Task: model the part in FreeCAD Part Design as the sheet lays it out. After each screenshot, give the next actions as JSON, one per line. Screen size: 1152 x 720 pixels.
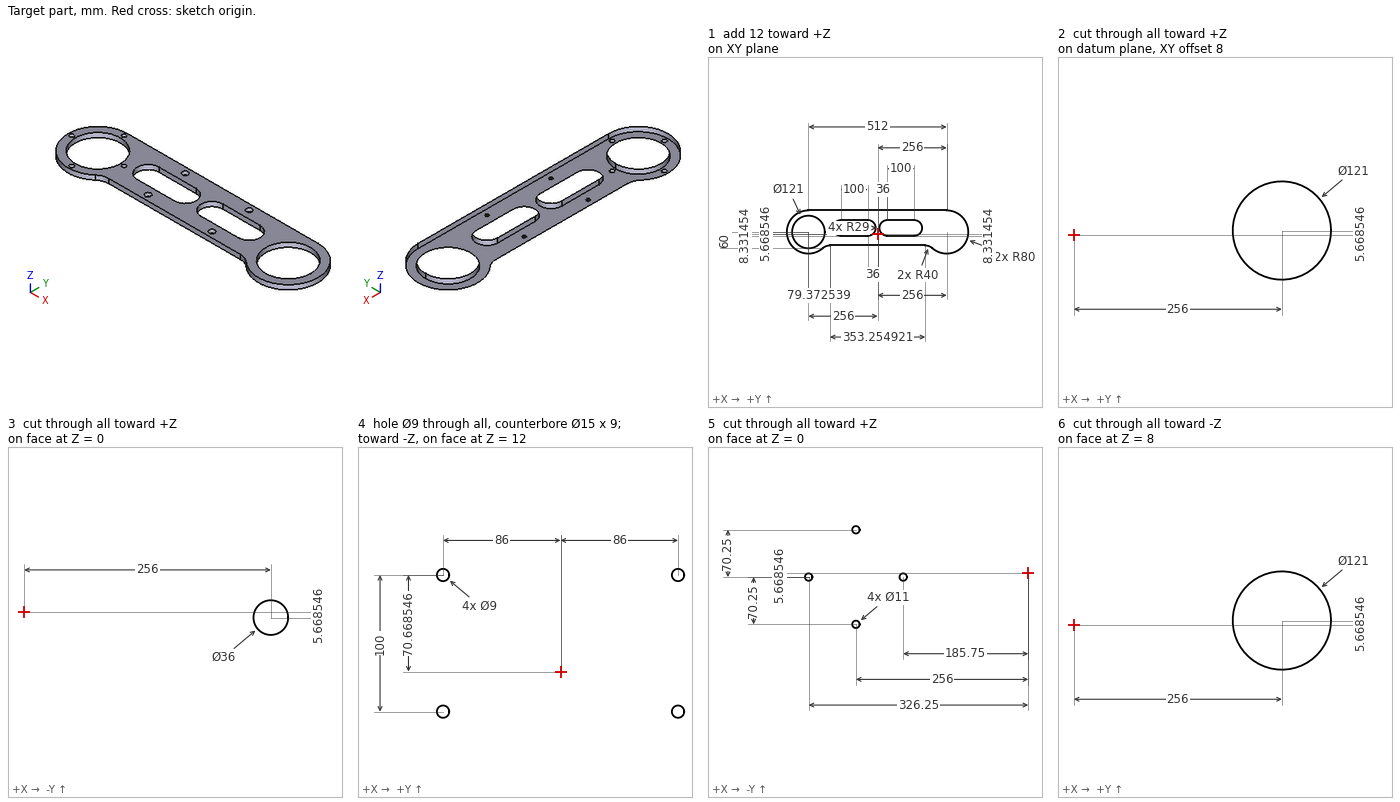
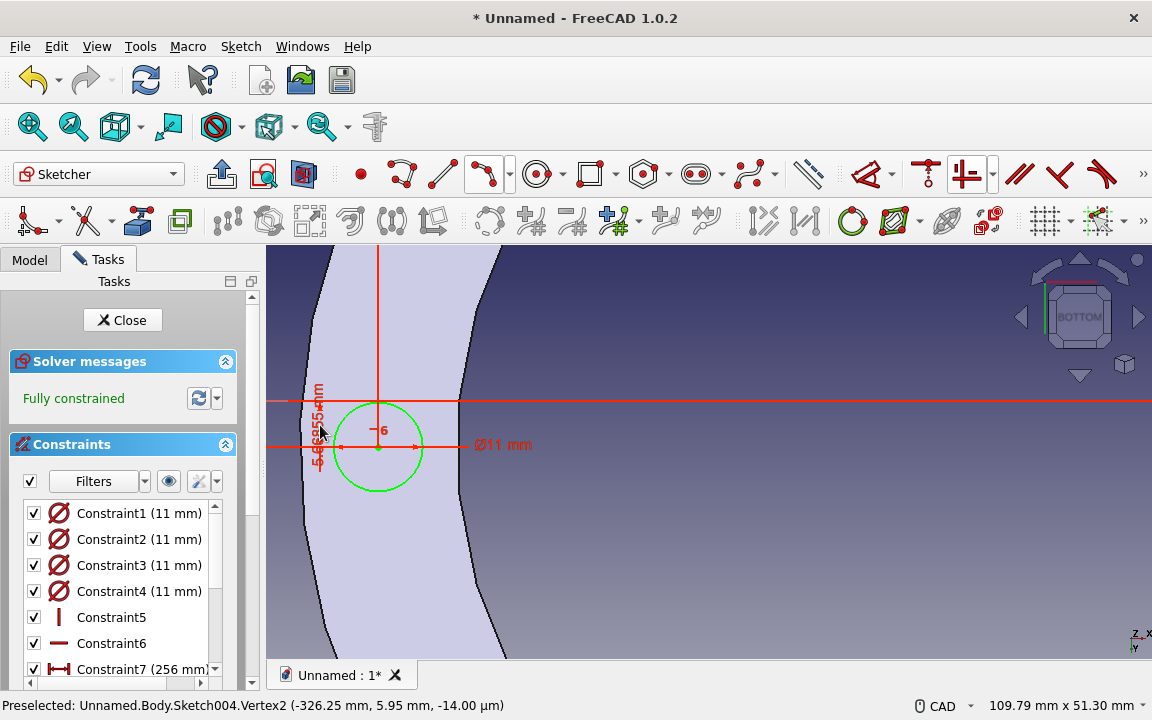
{"action": "left_click", "coordinate": [123, 320]}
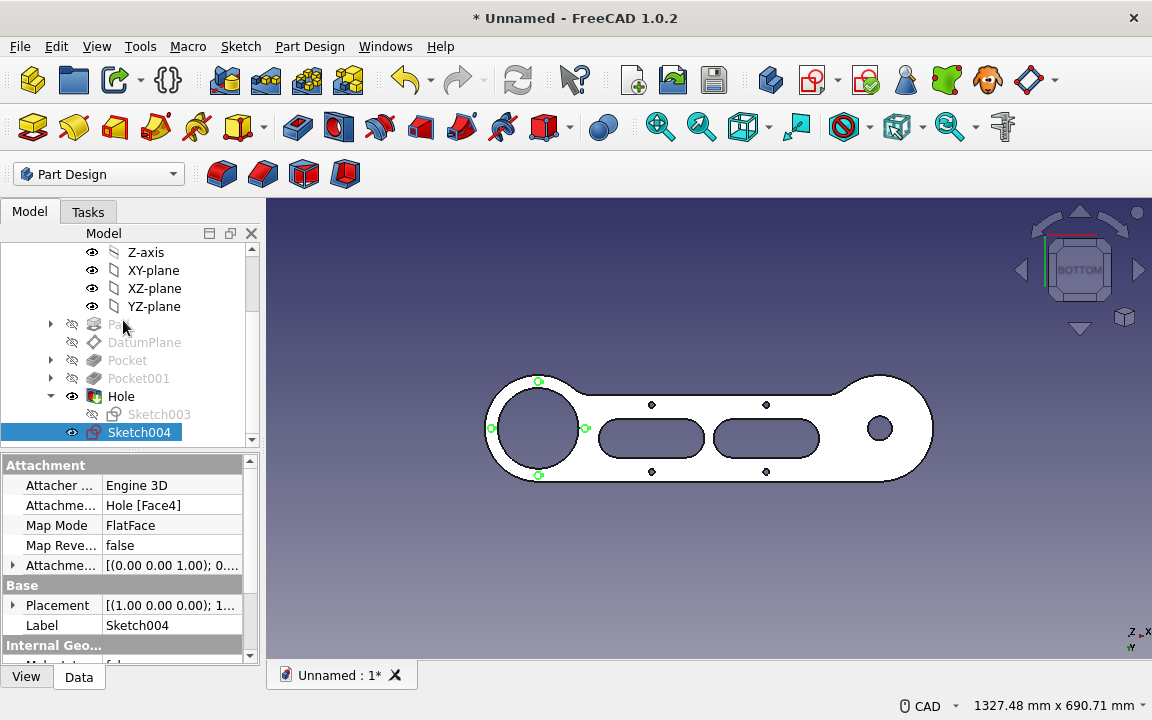
{"action": "left_click", "coordinate": [298, 128]}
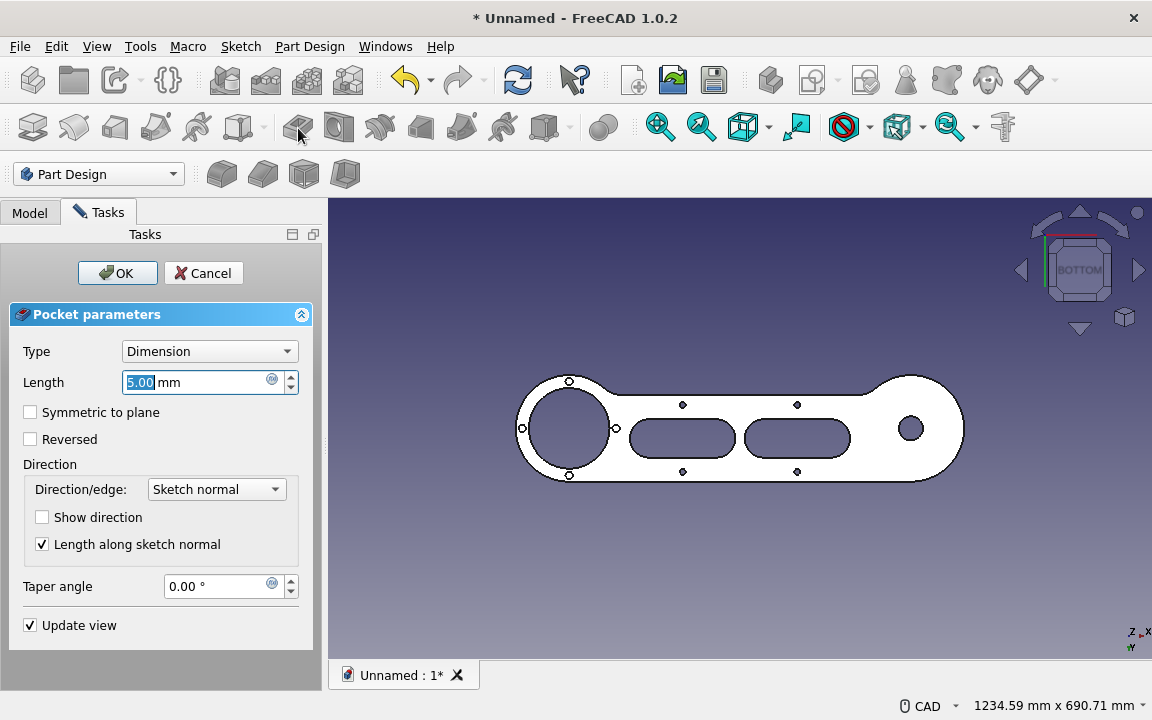
{"action": "left_click", "coordinate": [210, 352]}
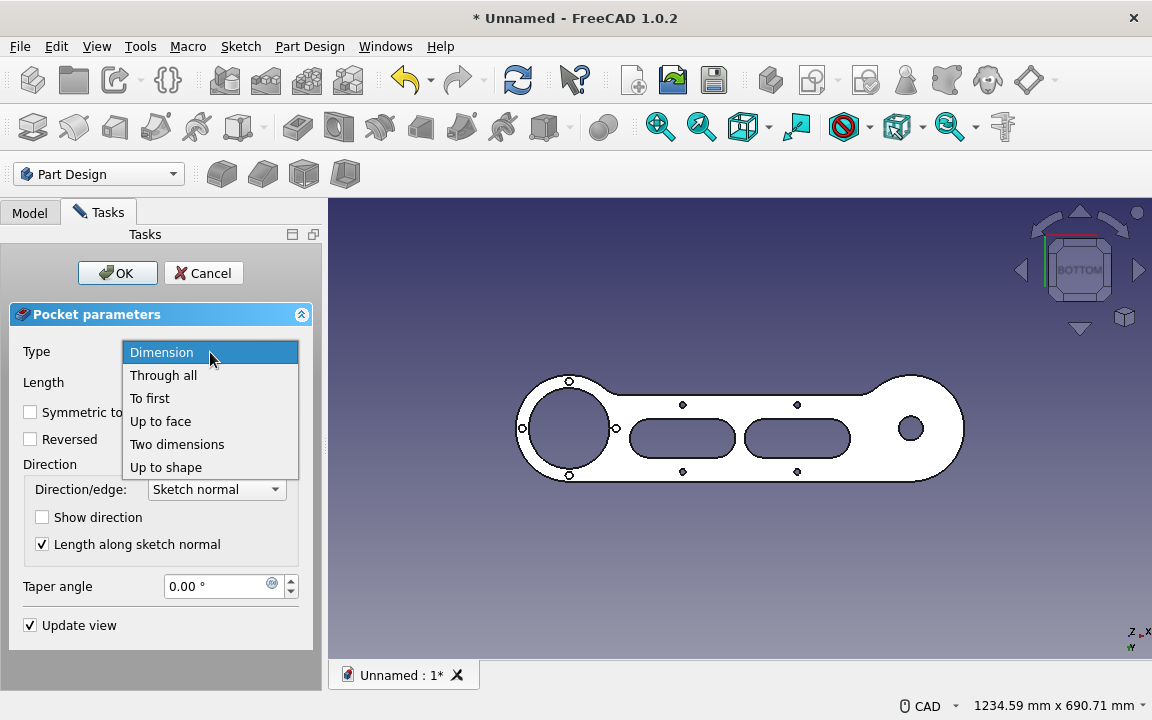
{"action": "left_click", "coordinate": [208, 376]}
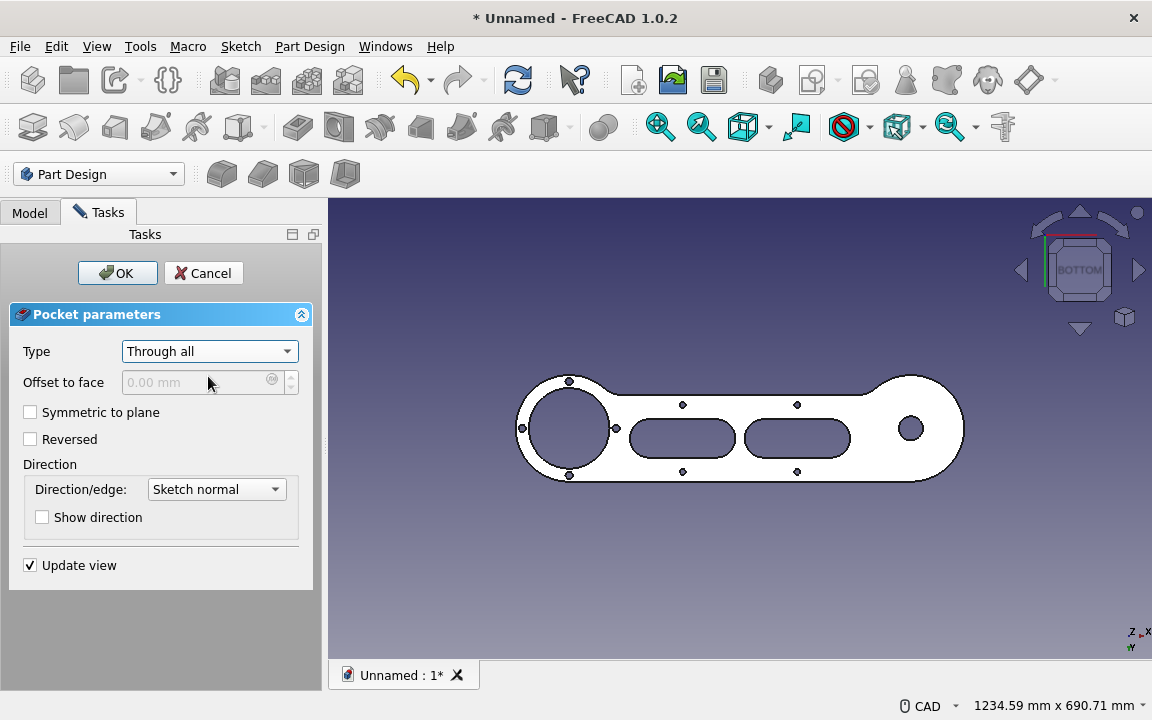
{"action": "left_click", "coordinate": [118, 273]}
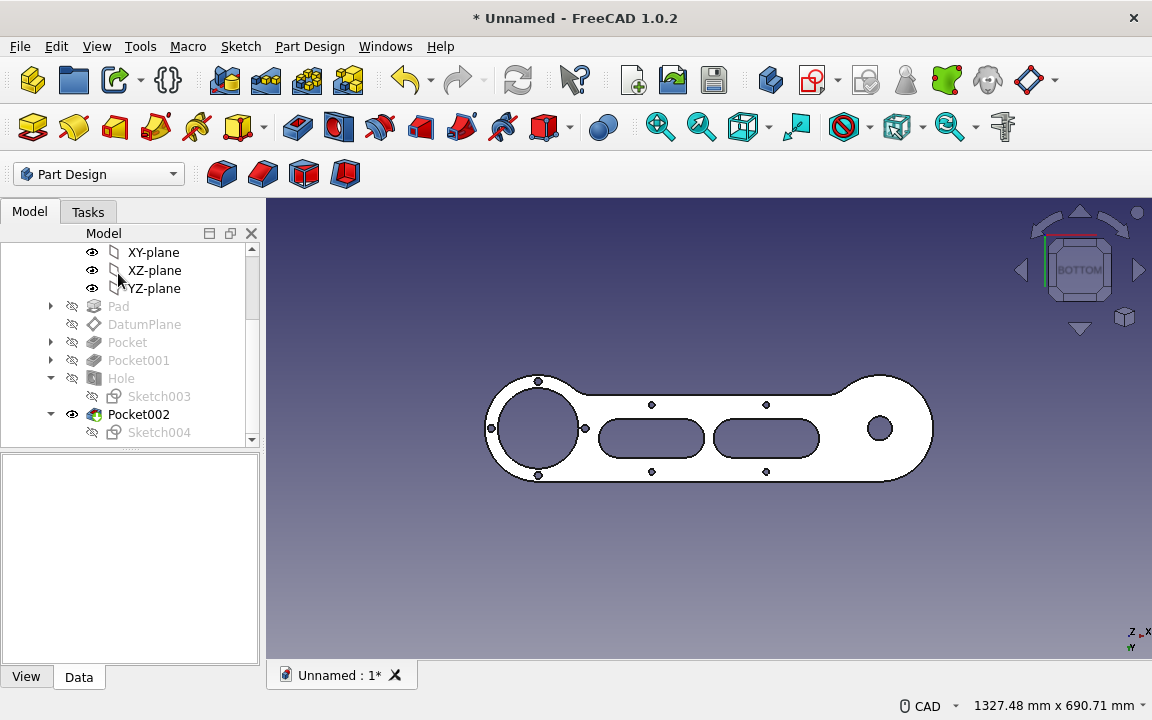
{"action": "key", "text": "0"}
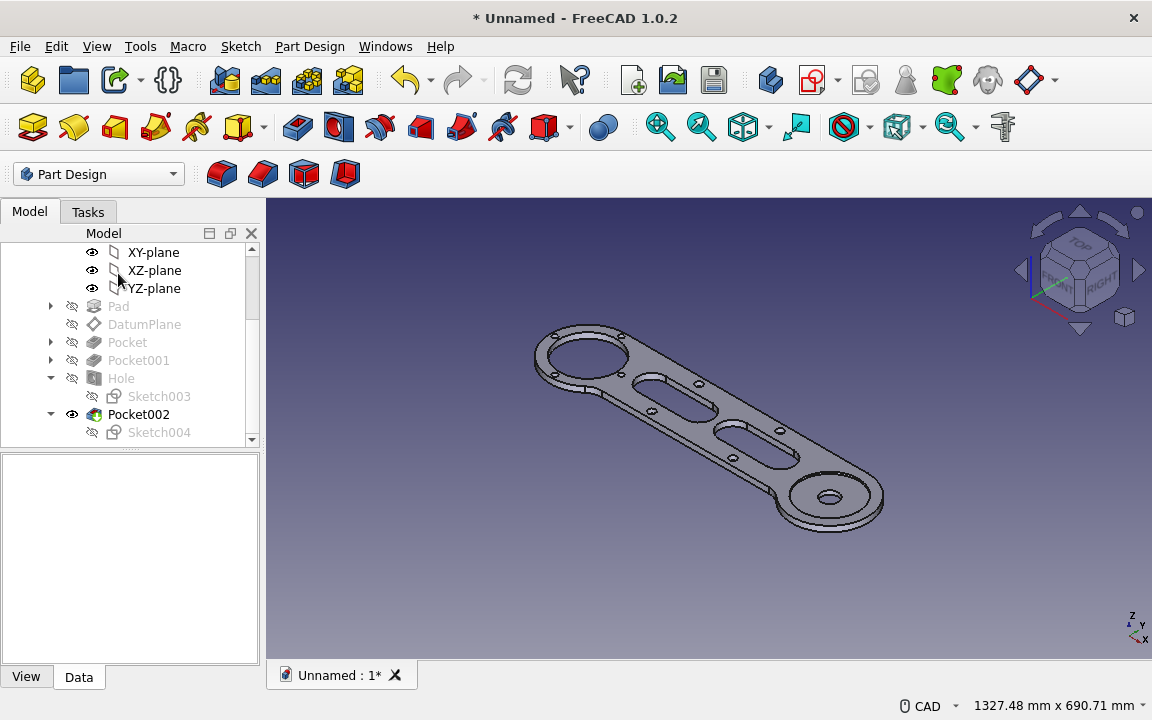
{"action": "left_click", "coordinate": [854, 491]}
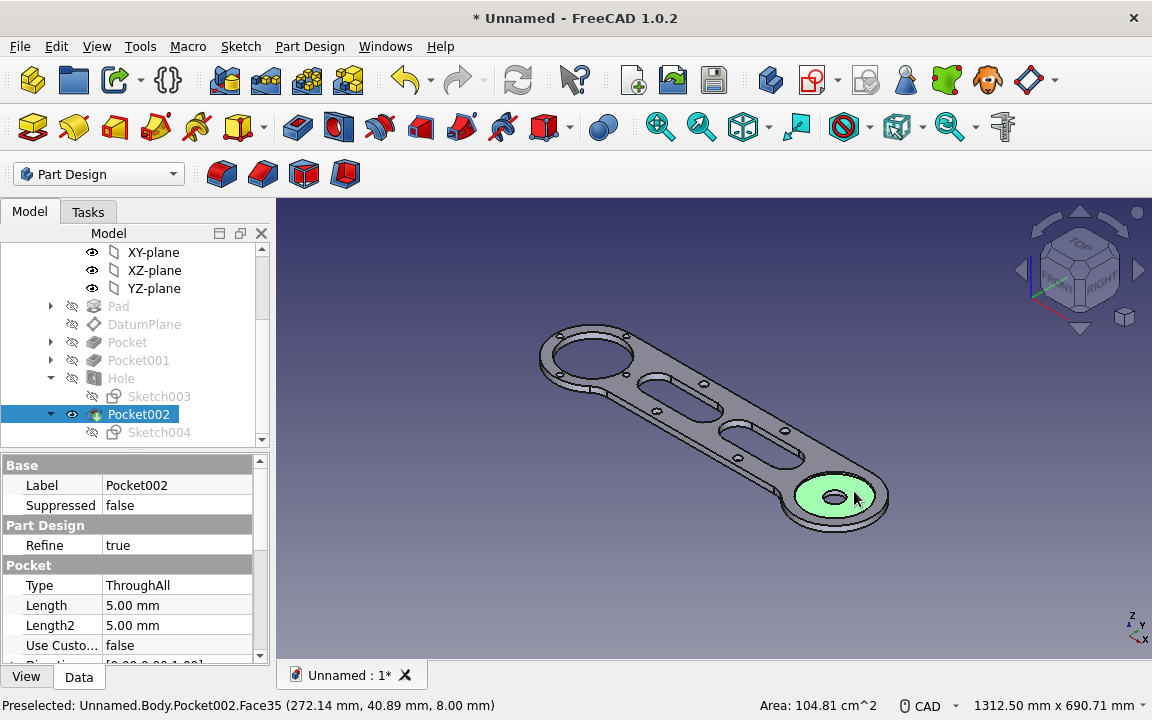
{"action": "left_click", "coordinate": [812, 80]}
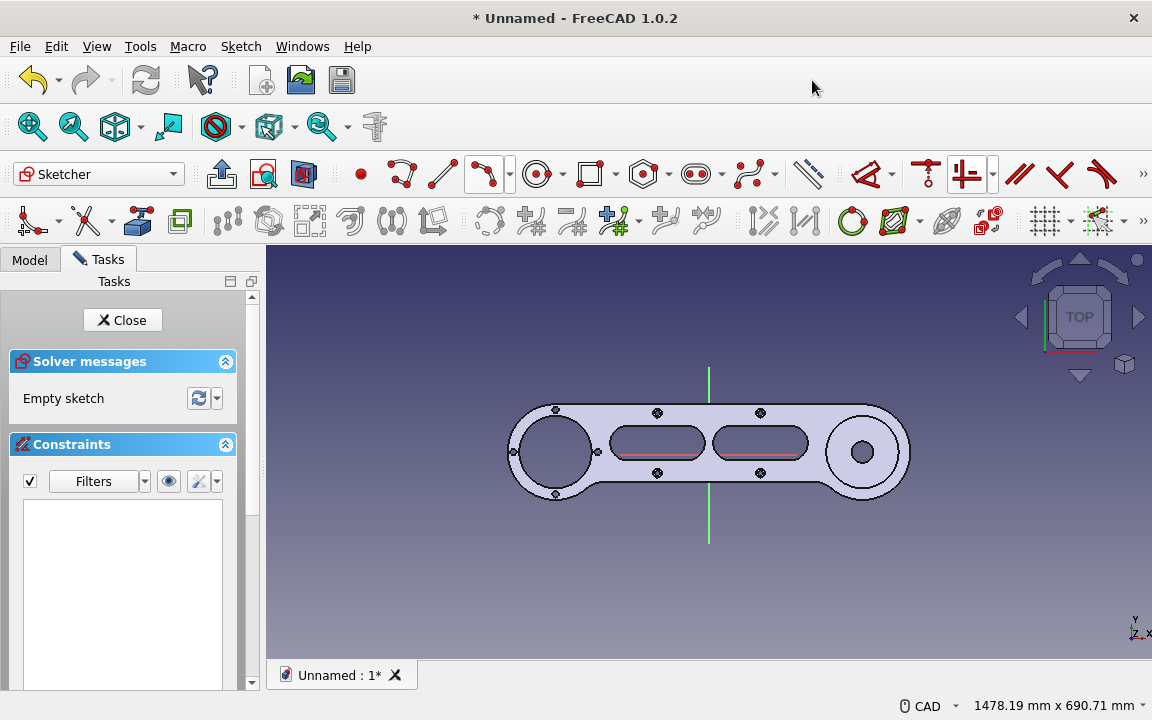
{"action": "left_click", "coordinate": [304, 174]}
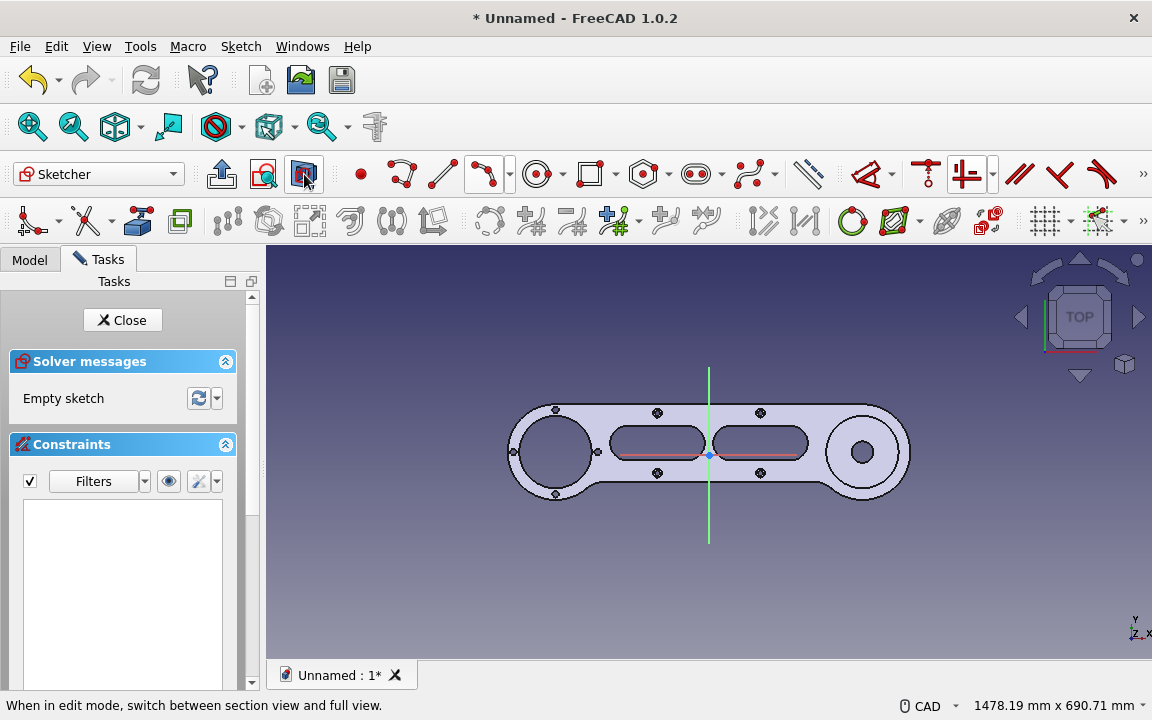
{"action": "scroll", "coordinate": [958, 452], "scroll_direction": "up", "scroll_amount": 6}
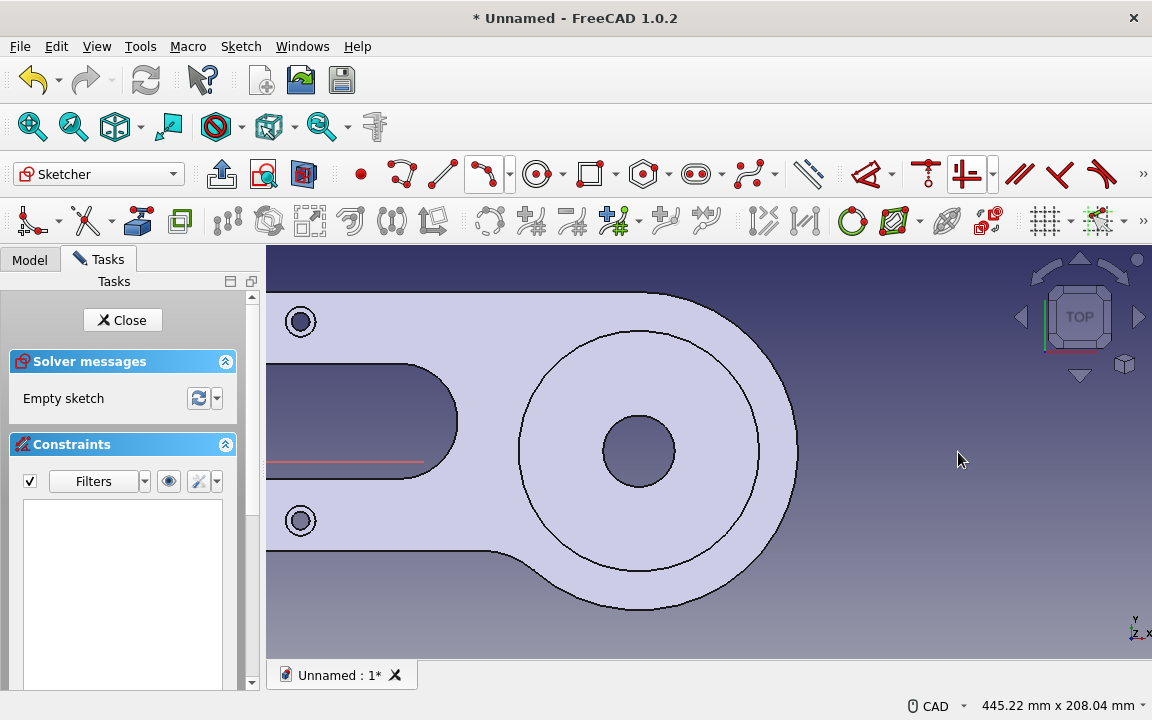
{"action": "left_click", "coordinate": [536, 174]}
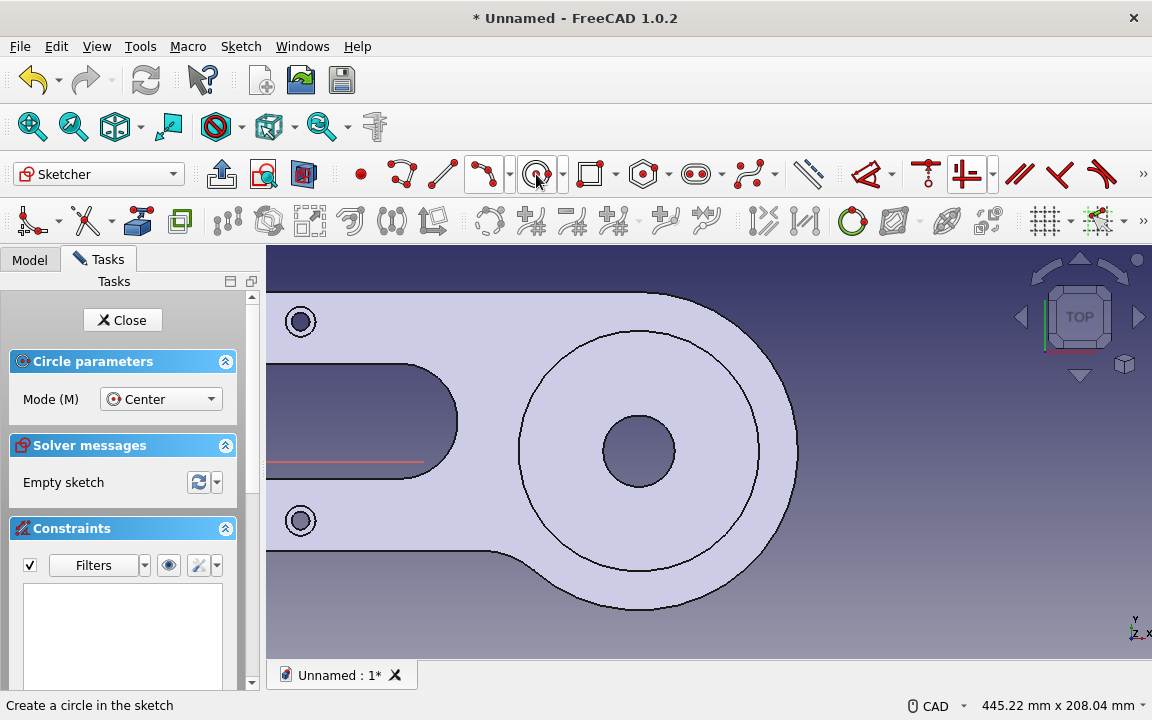
{"action": "scroll", "coordinate": [639, 451], "scroll_direction": "up", "scroll_amount": 2}